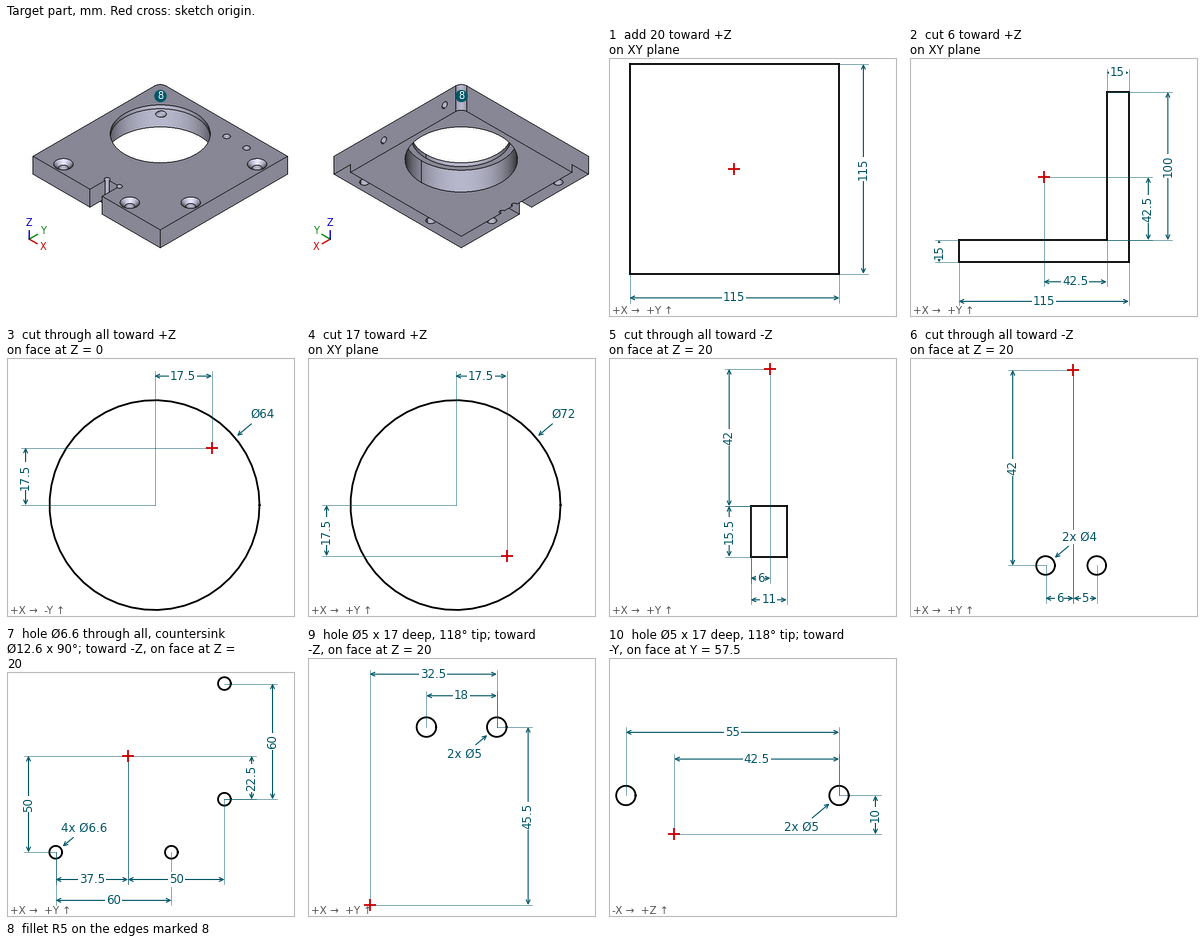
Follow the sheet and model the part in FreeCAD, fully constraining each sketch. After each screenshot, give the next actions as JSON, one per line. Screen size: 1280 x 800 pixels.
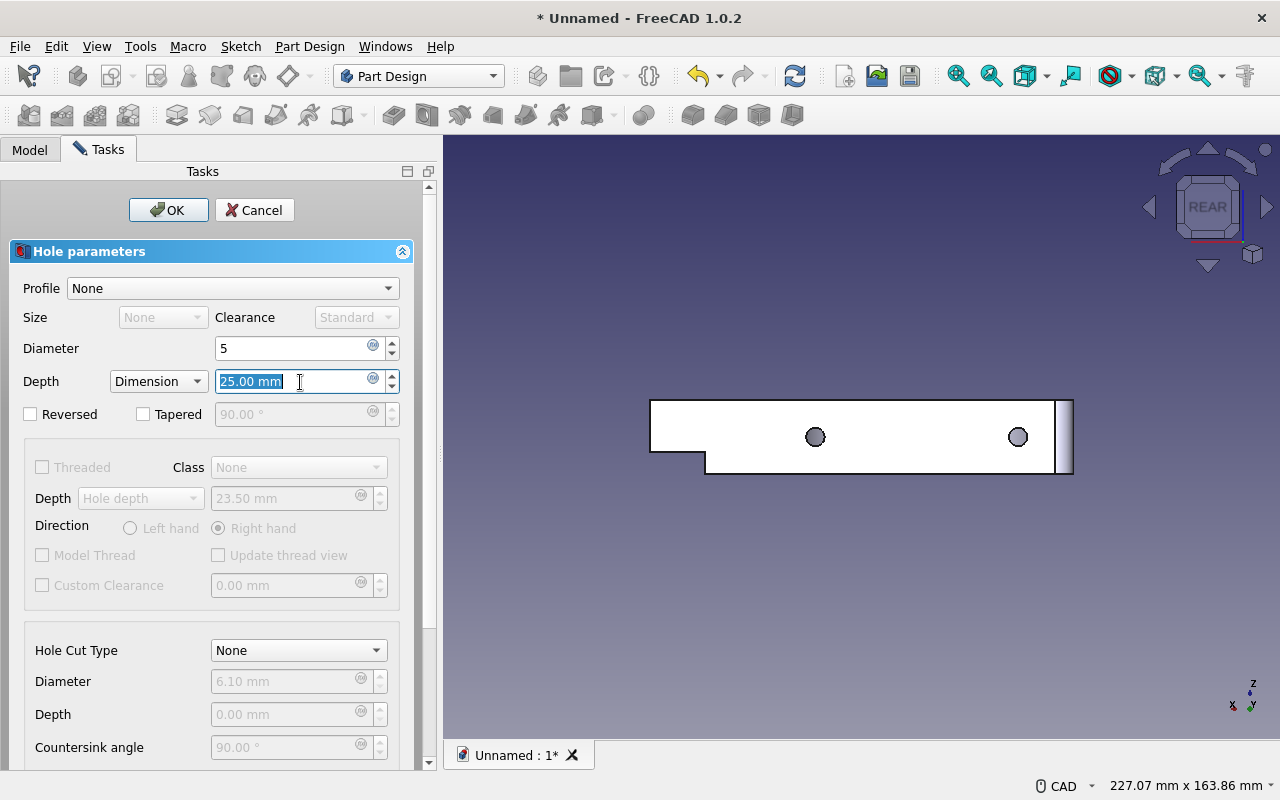
{"action": "type", "text": "17"}
{"action": "key", "text": "Tab"}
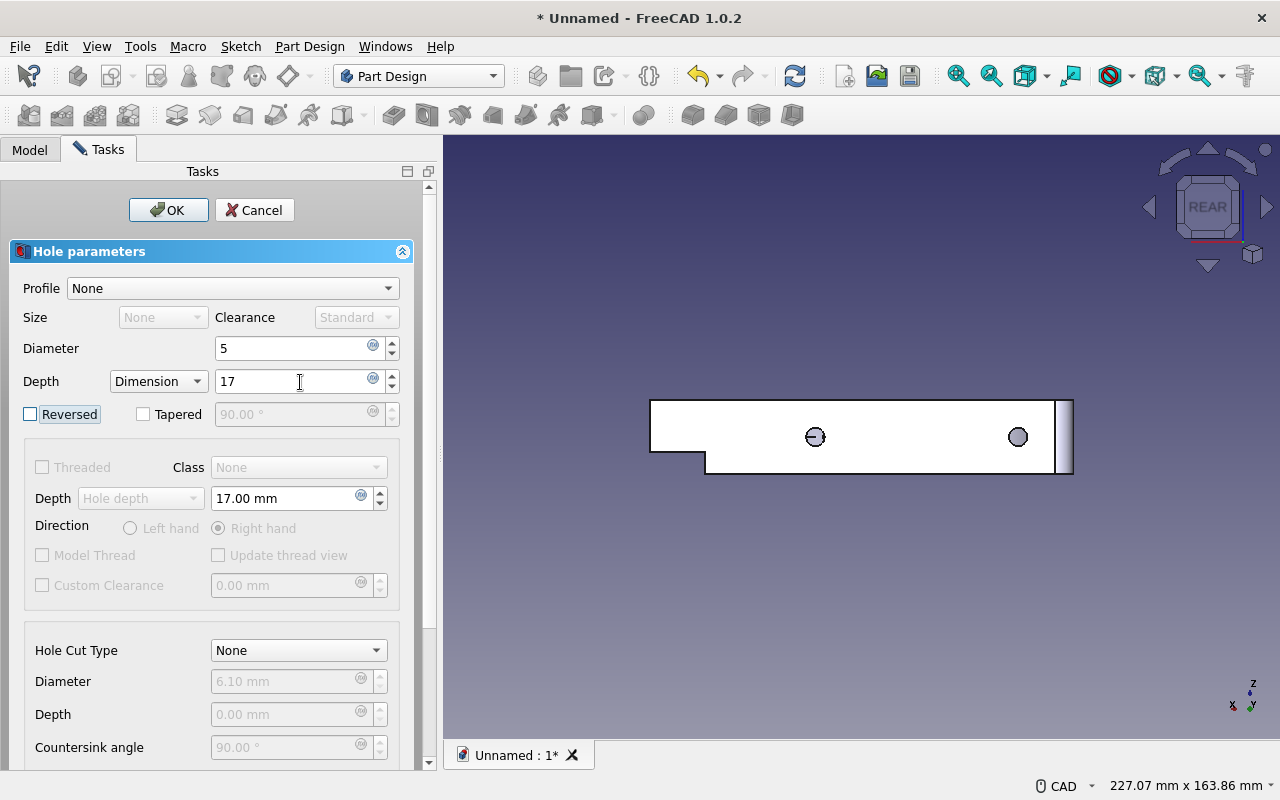
{"action": "left_click", "coordinate": [169, 210]}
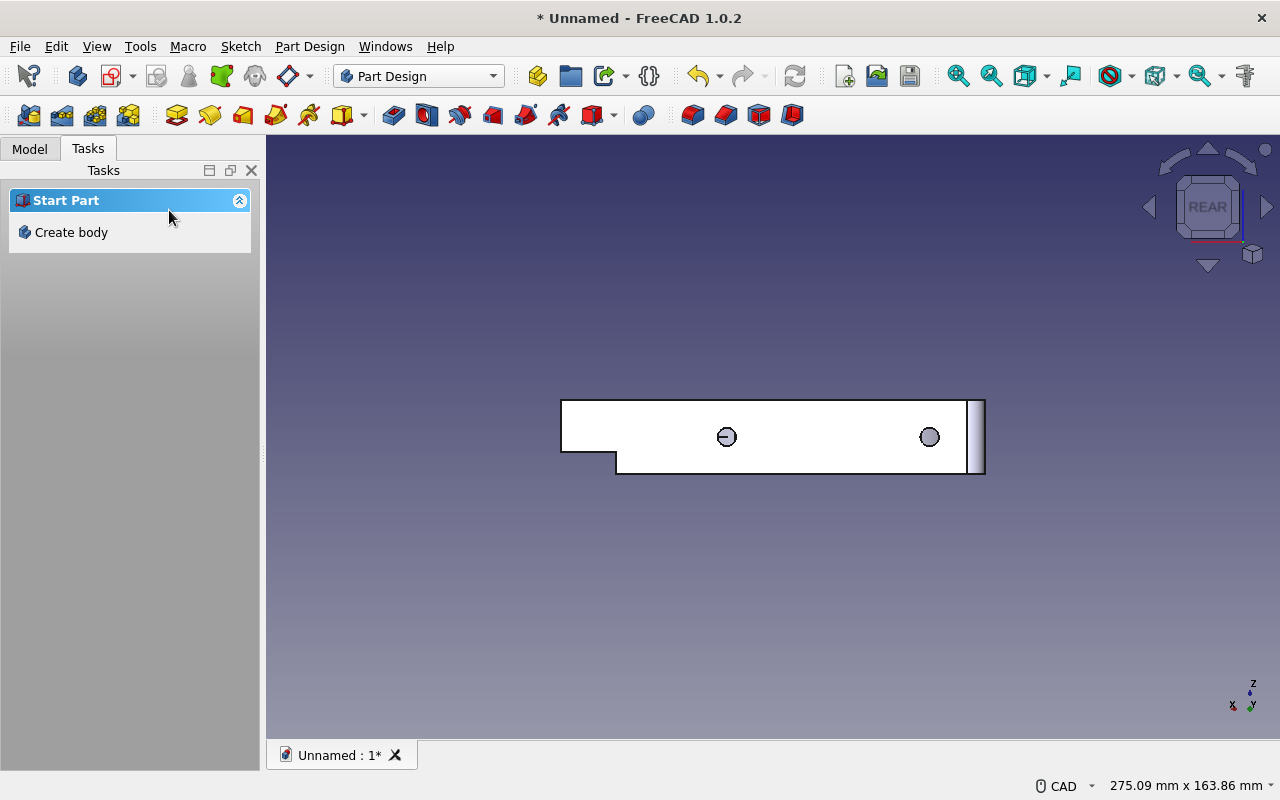
{"action": "key", "text": "0"}